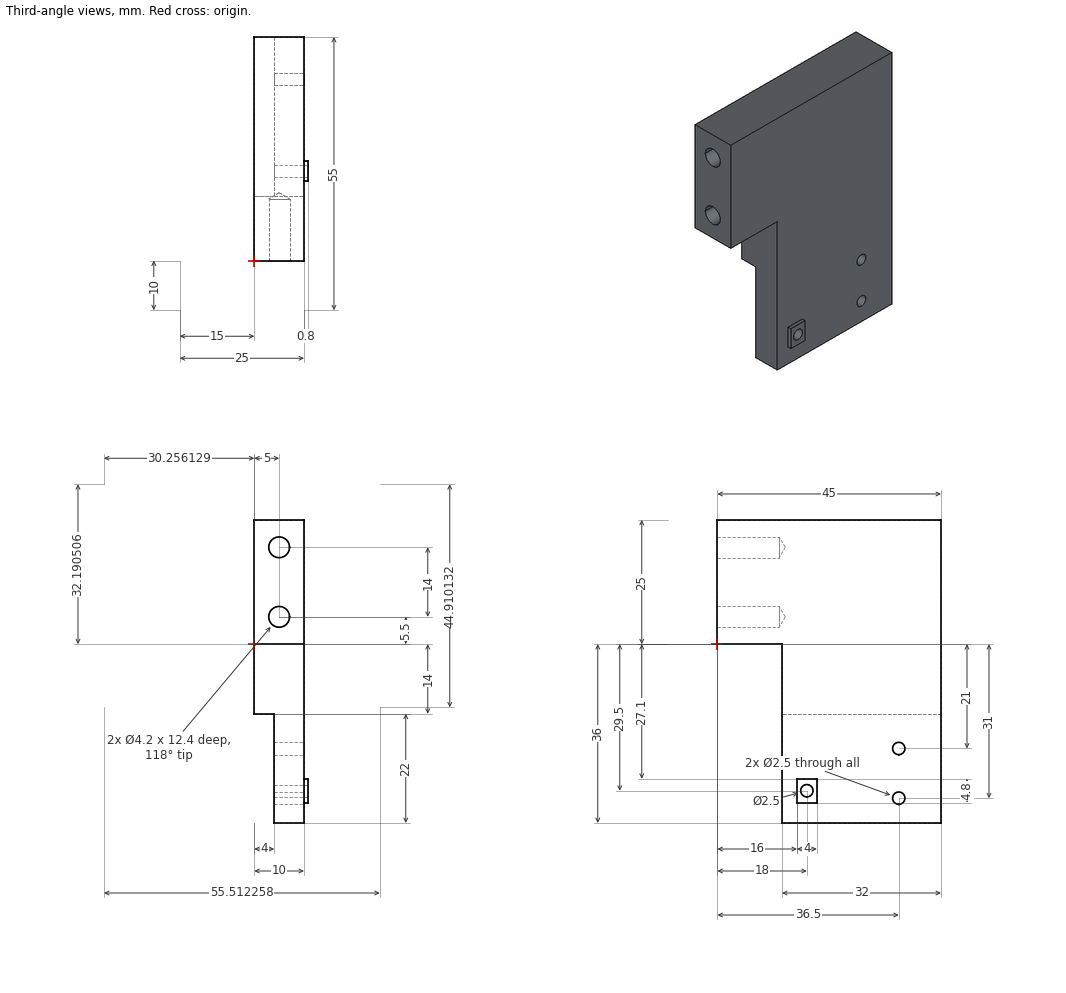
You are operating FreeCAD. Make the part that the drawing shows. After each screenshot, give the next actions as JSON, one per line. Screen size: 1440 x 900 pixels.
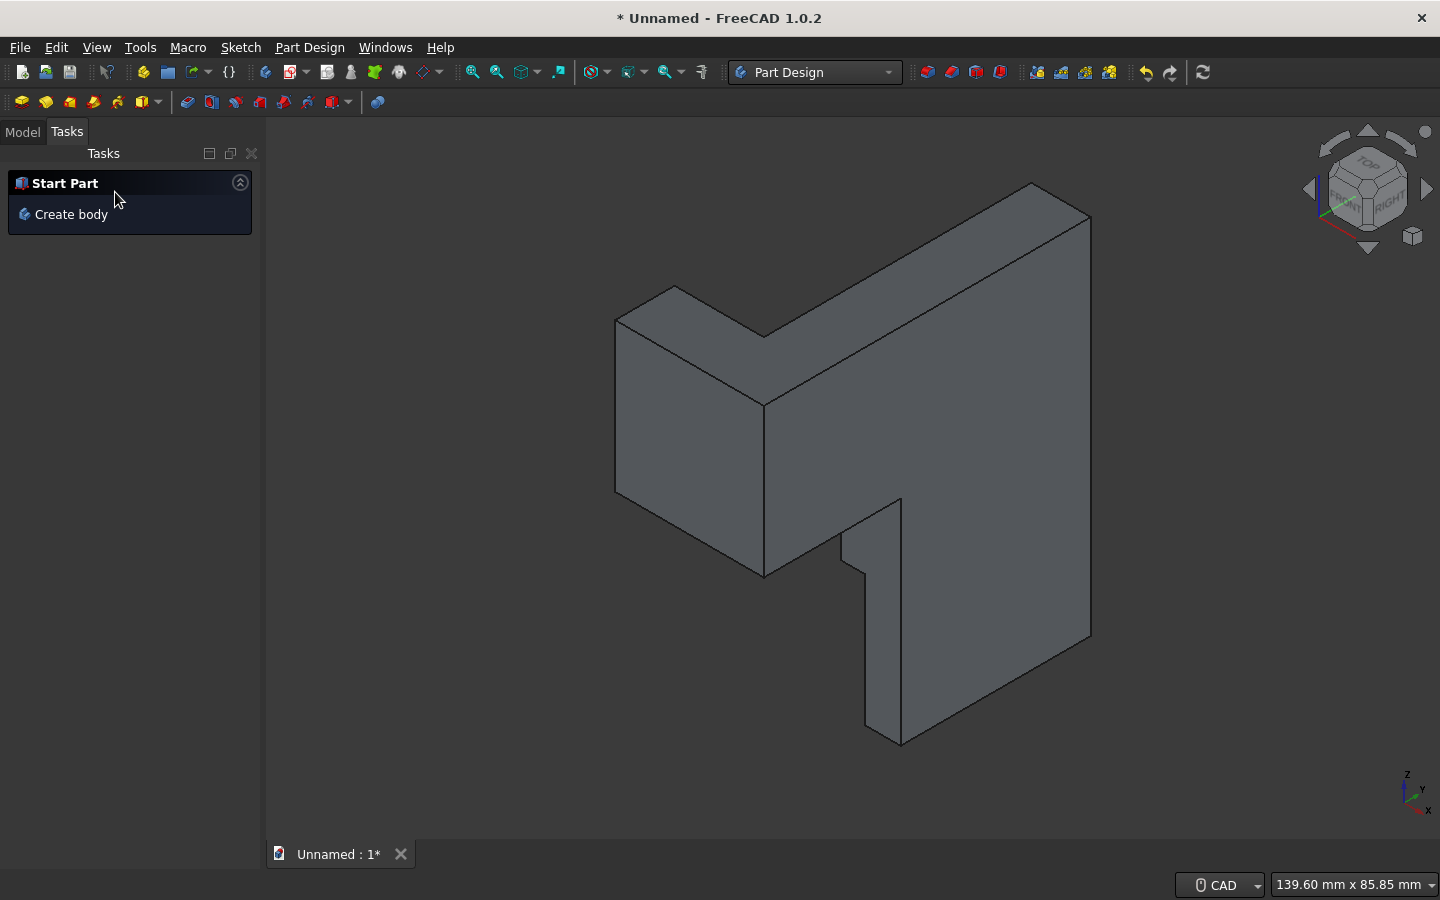
{"action": "left_click", "coordinate": [689, 448]}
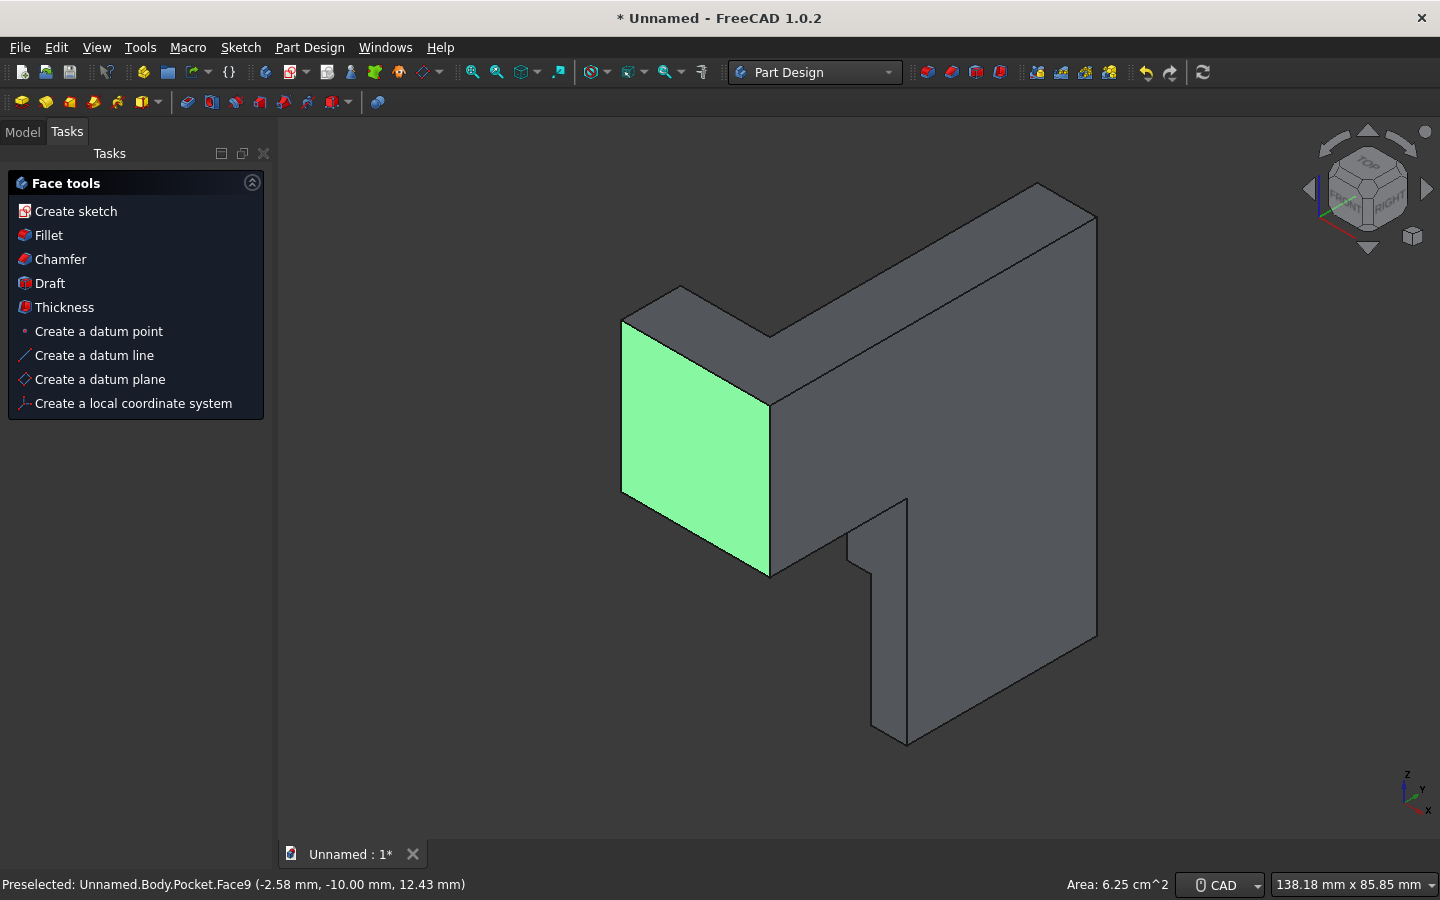
{"action": "left_click", "coordinate": [290, 72]}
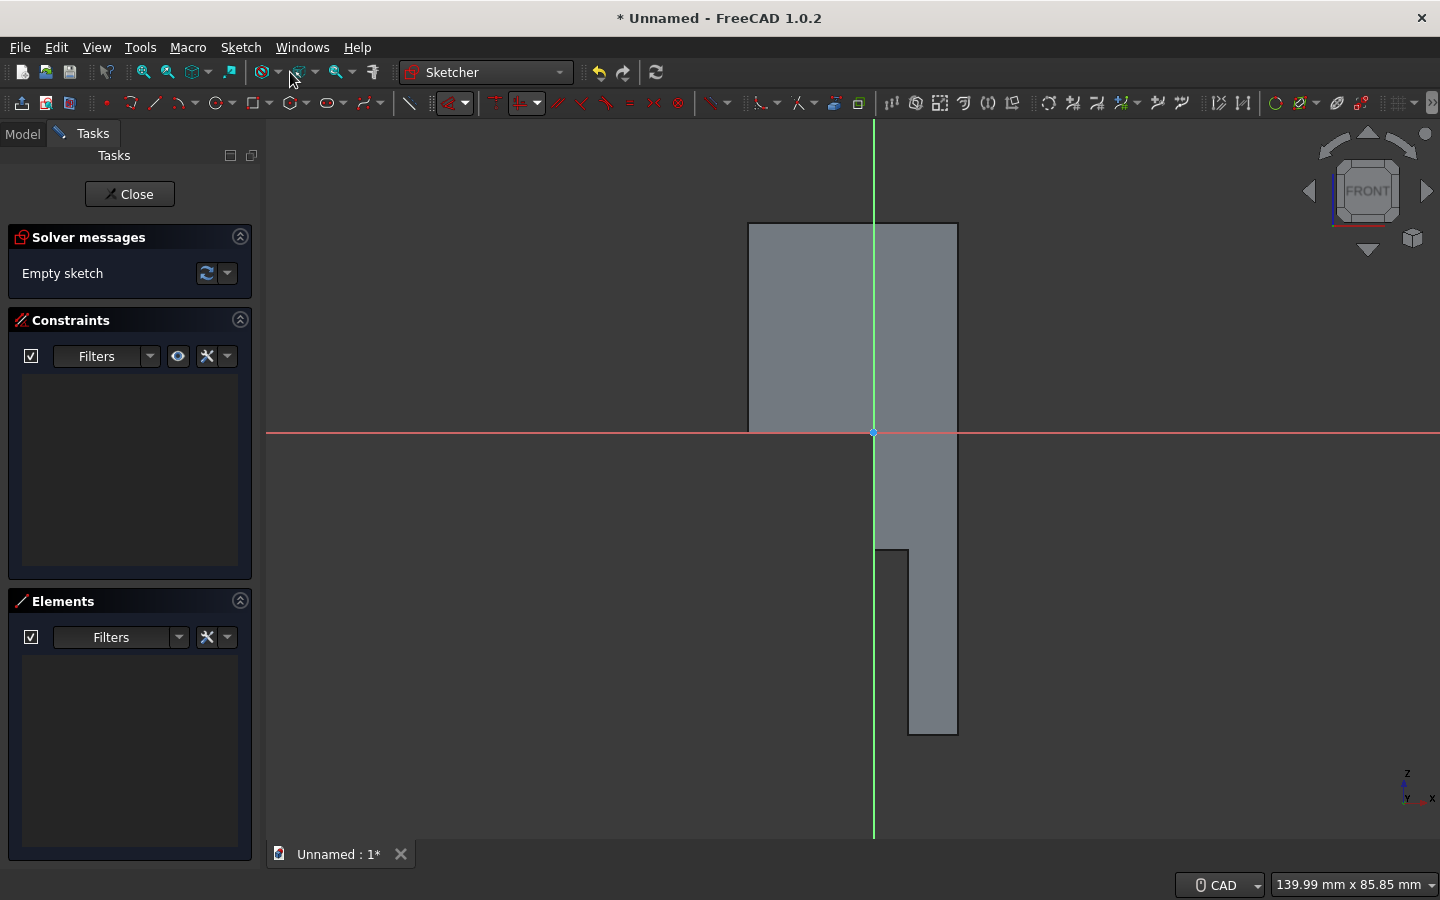
{"action": "scroll", "coordinate": [475, 811], "scroll_direction": "down", "scroll_amount": 1}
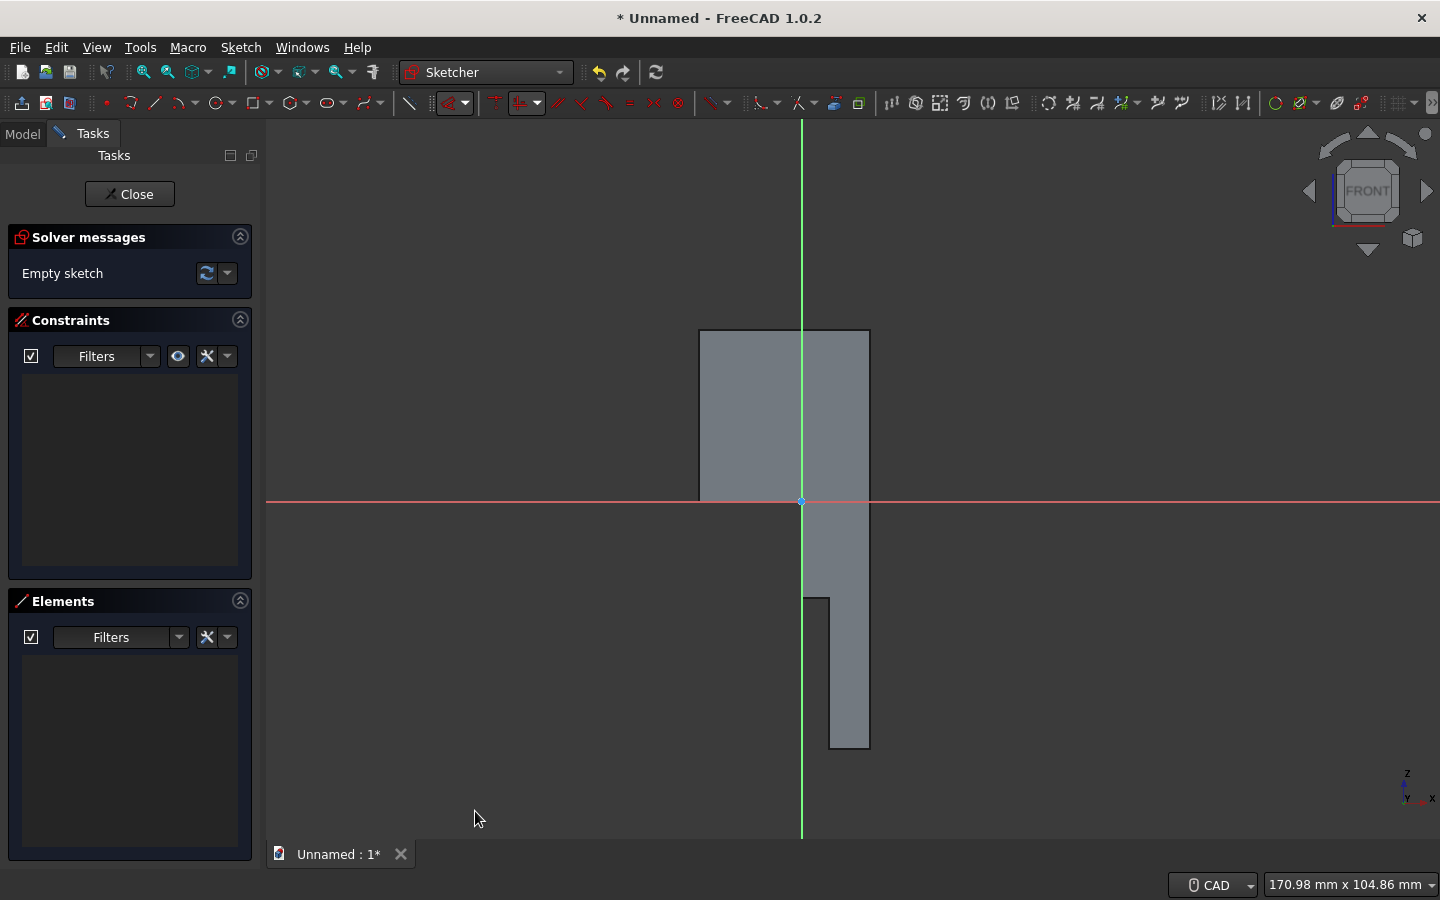
{"action": "scroll", "coordinate": [785, 345], "scroll_direction": "up", "scroll_amount": 2}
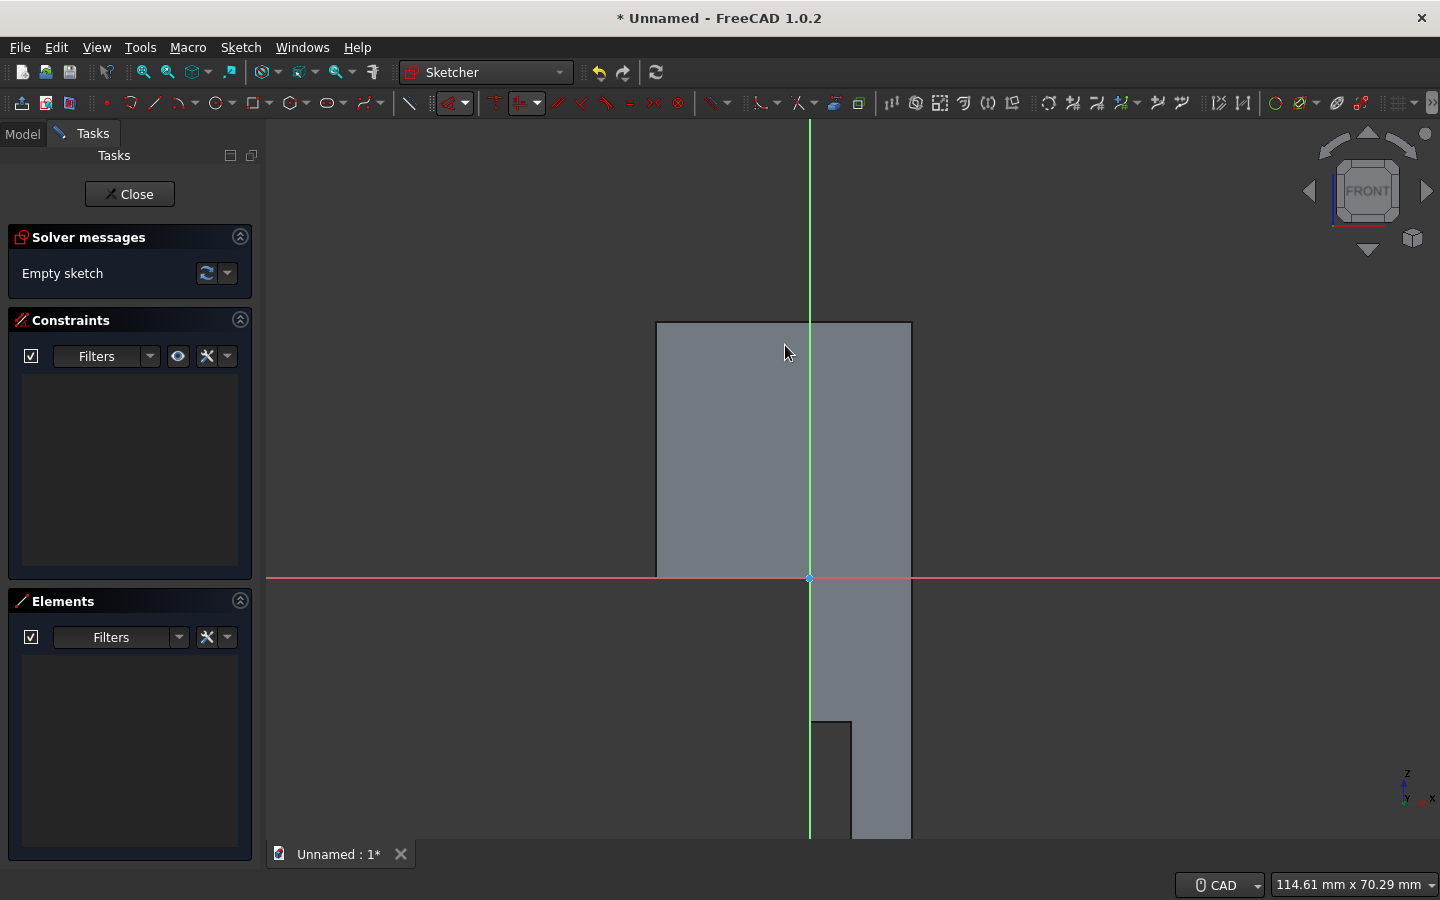
{"action": "key", "text": "g r"}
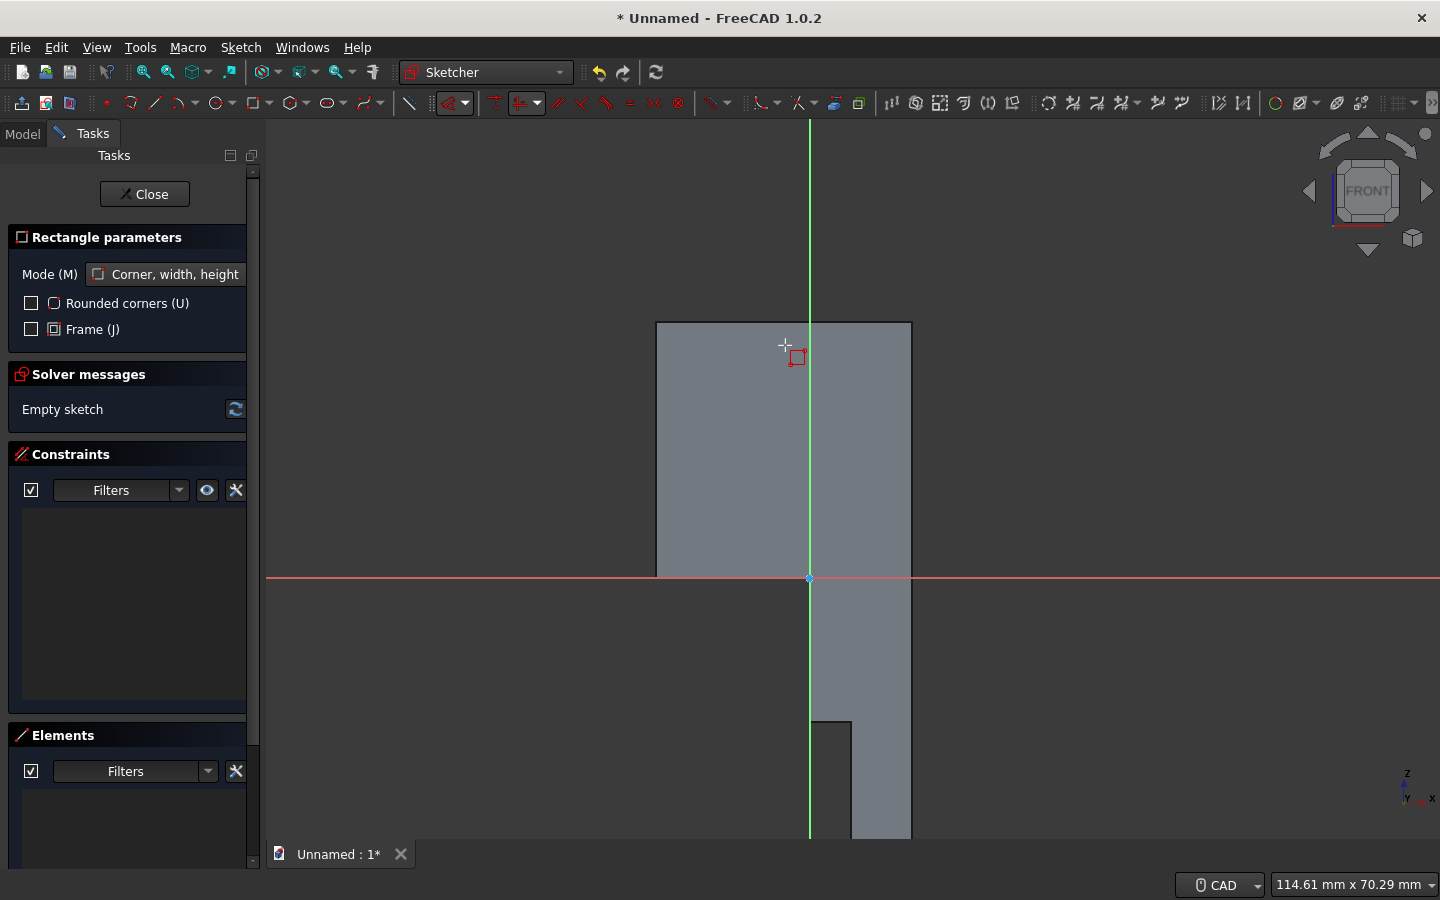
{"action": "left_click", "coordinate": [500, 249]}
{"action": "mouse_move", "coordinate": [1068, 709]}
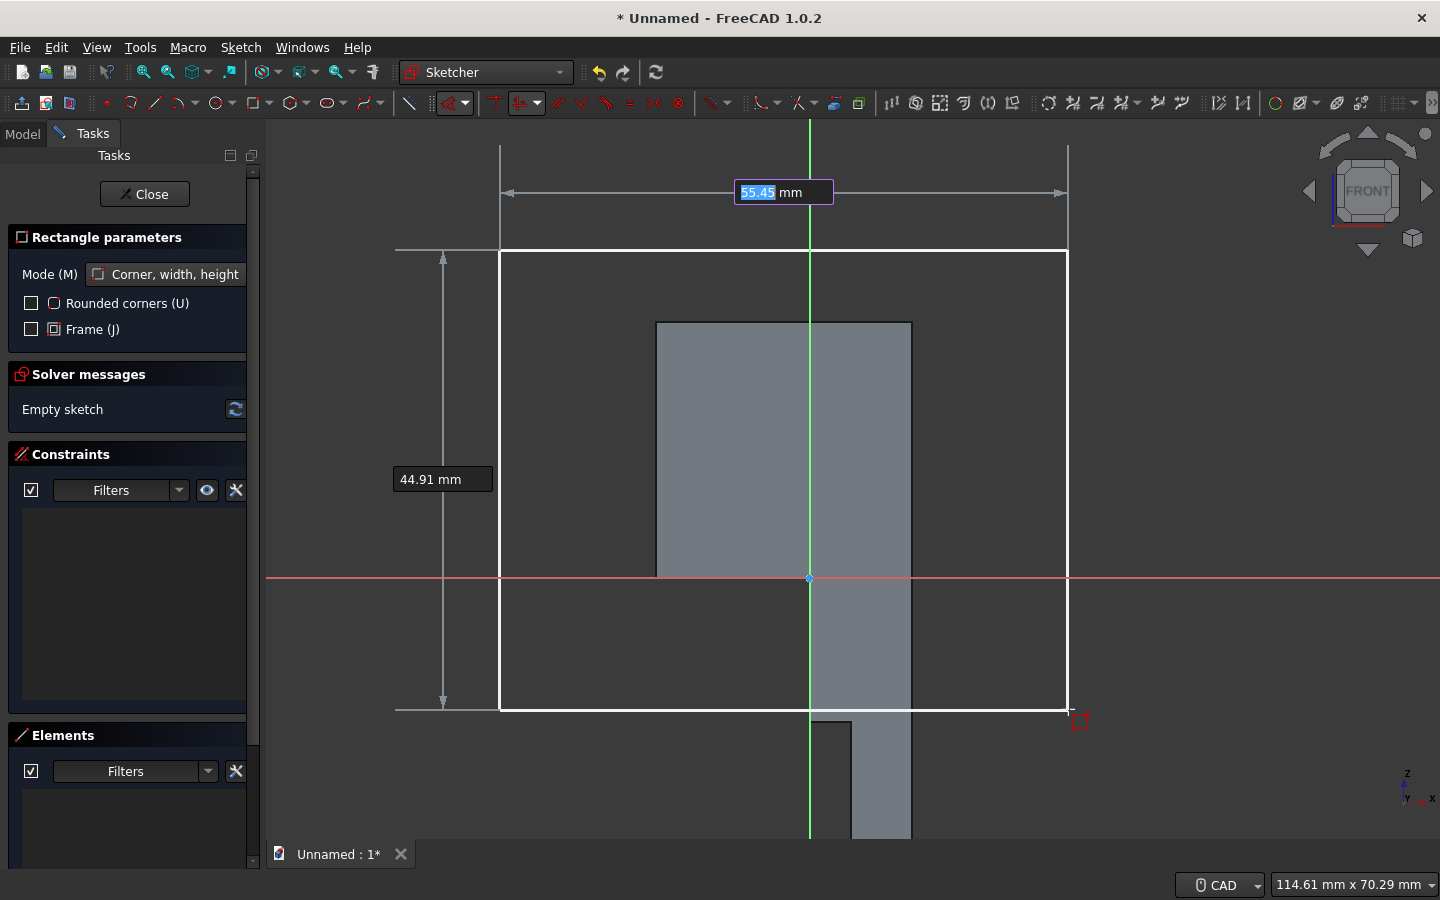
{"action": "type", "text": "55.512258"}
{"action": "key", "text": "Tab"}
{"action": "type", "text": "44.910132"}
{"action": "key", "text": "Return"}
{"action": "key", "text": "Escape"}